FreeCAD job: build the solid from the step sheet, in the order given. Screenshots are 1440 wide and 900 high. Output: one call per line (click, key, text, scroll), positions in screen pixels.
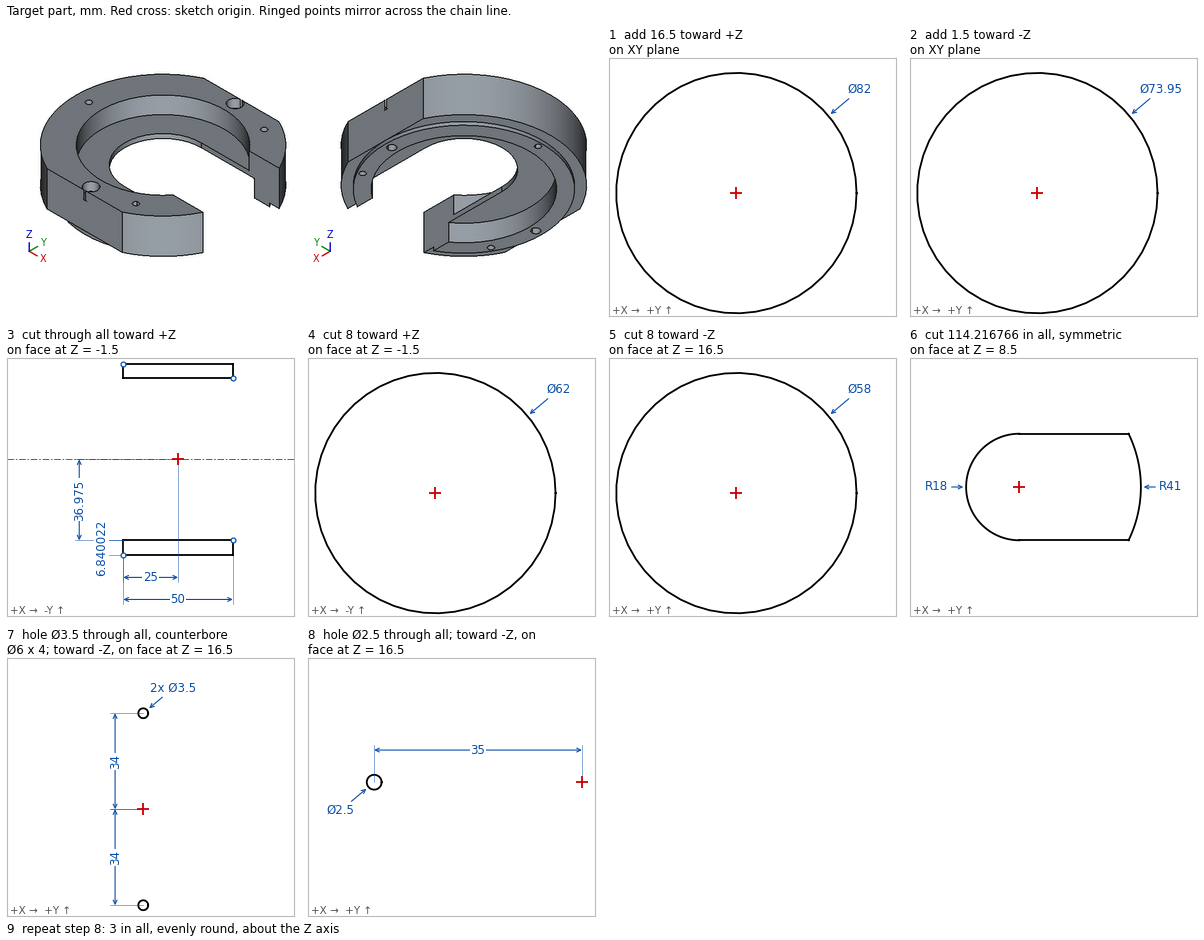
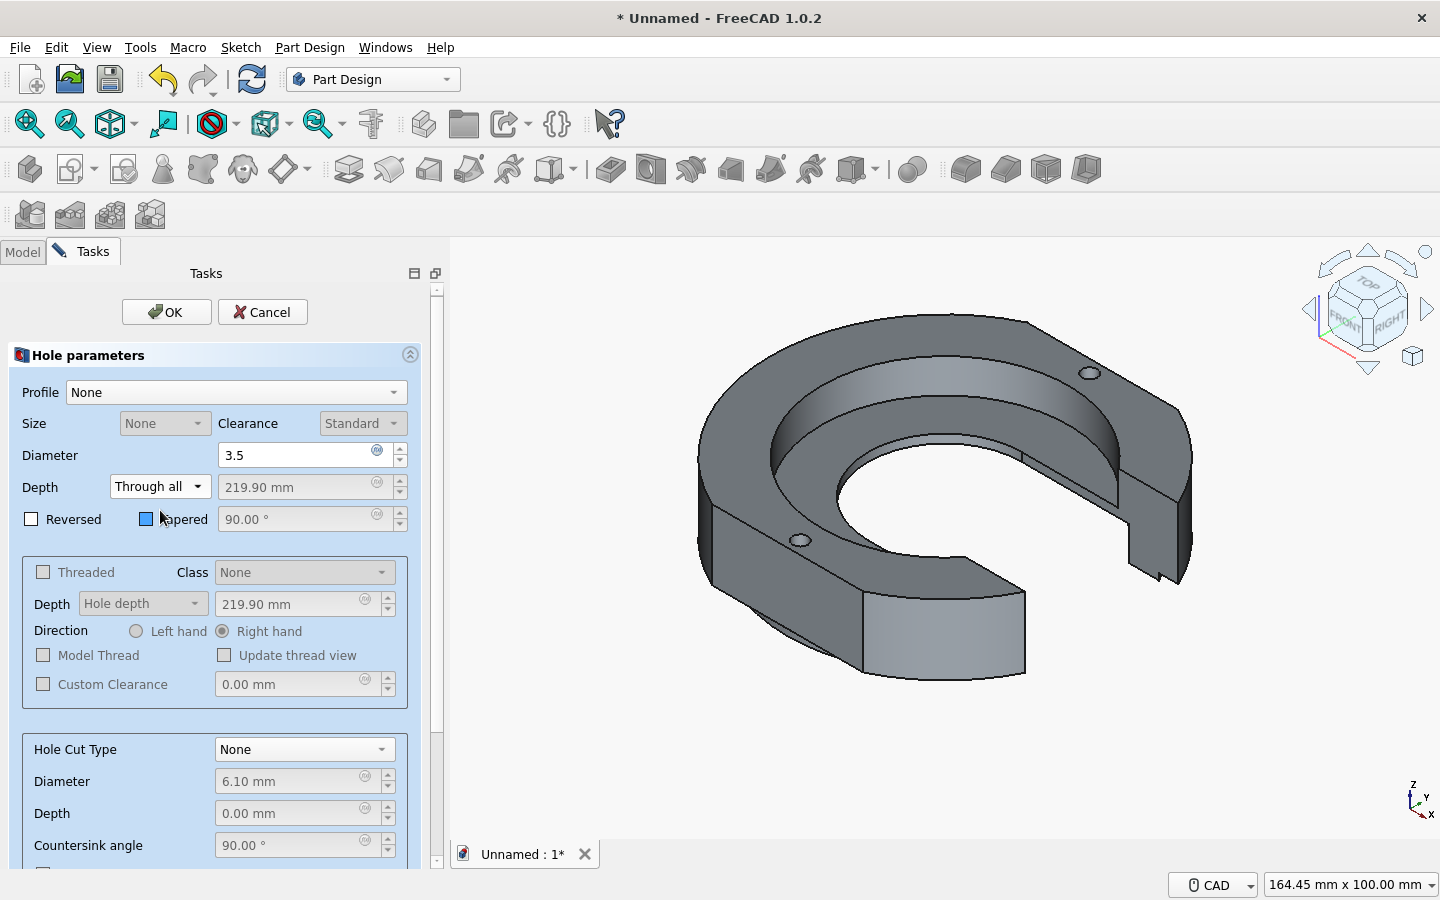
click(306, 750)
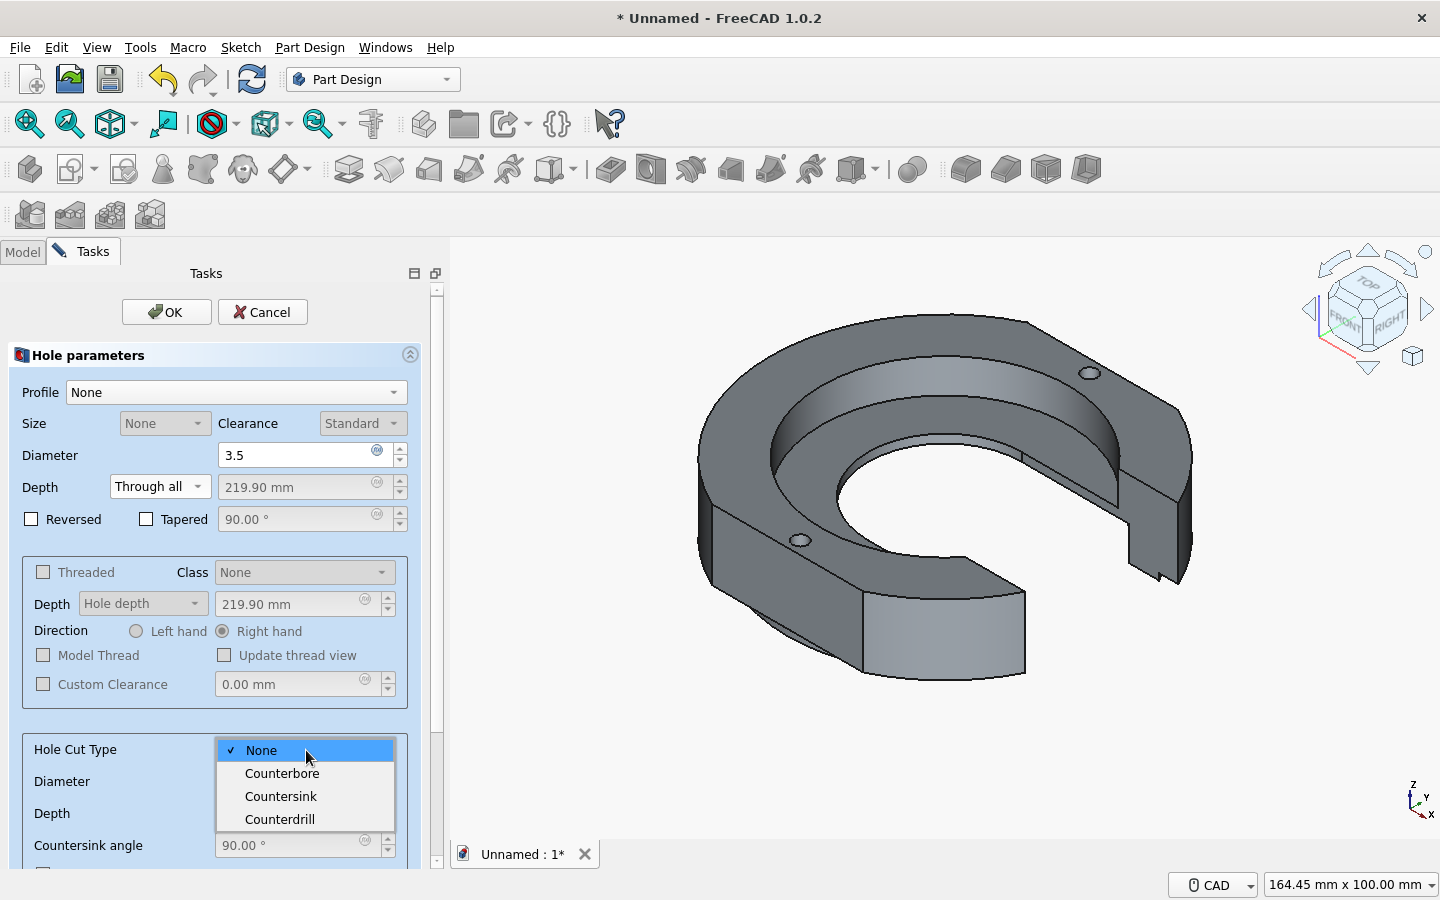
click(304, 774)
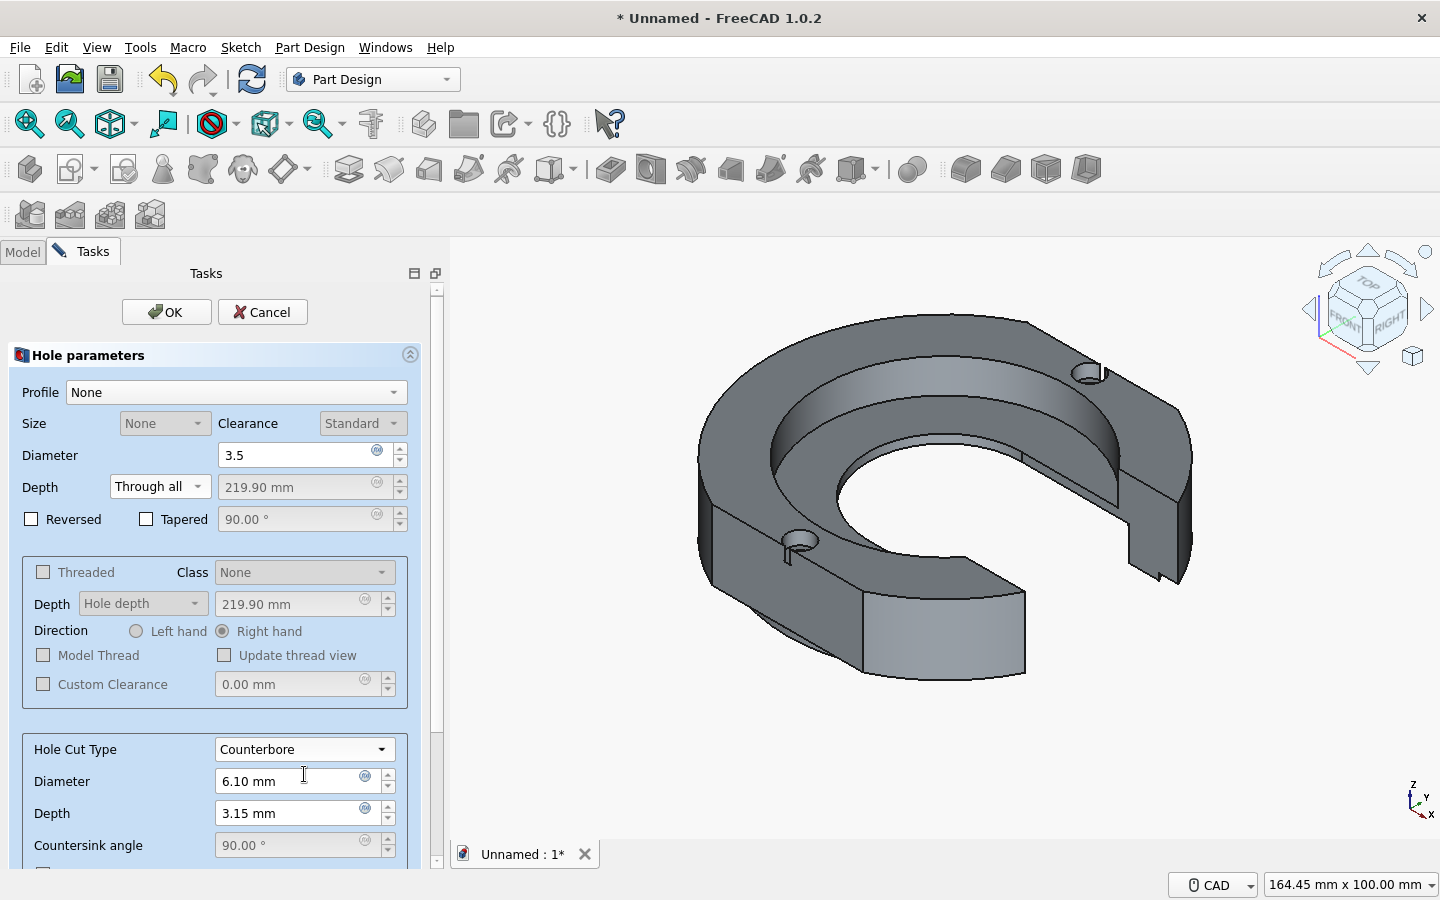
triple_click(298, 781)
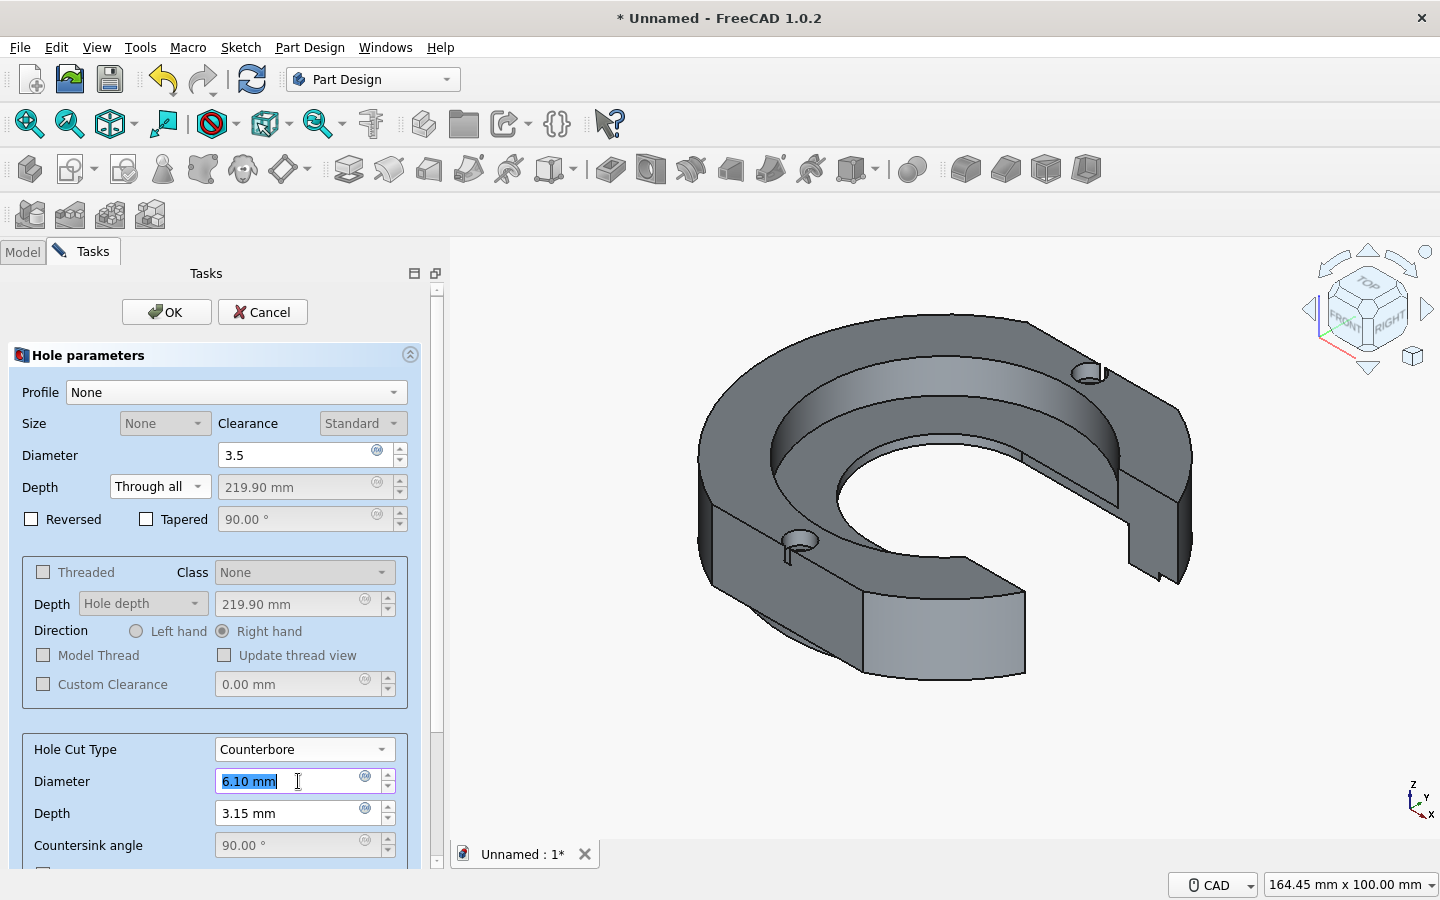
text(6)
key(Tab)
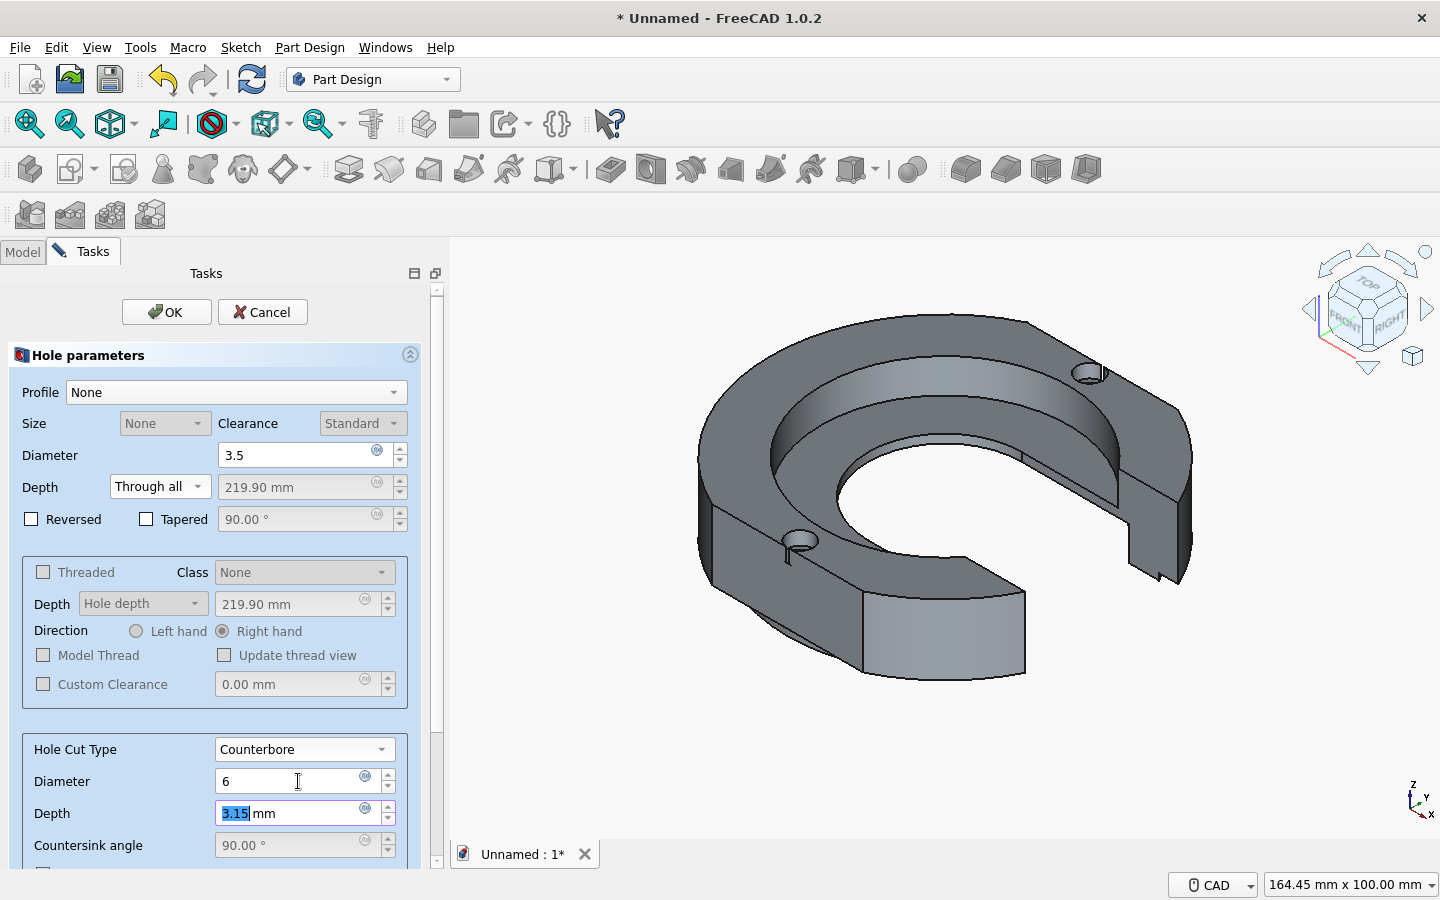
text(4)
key(Tab)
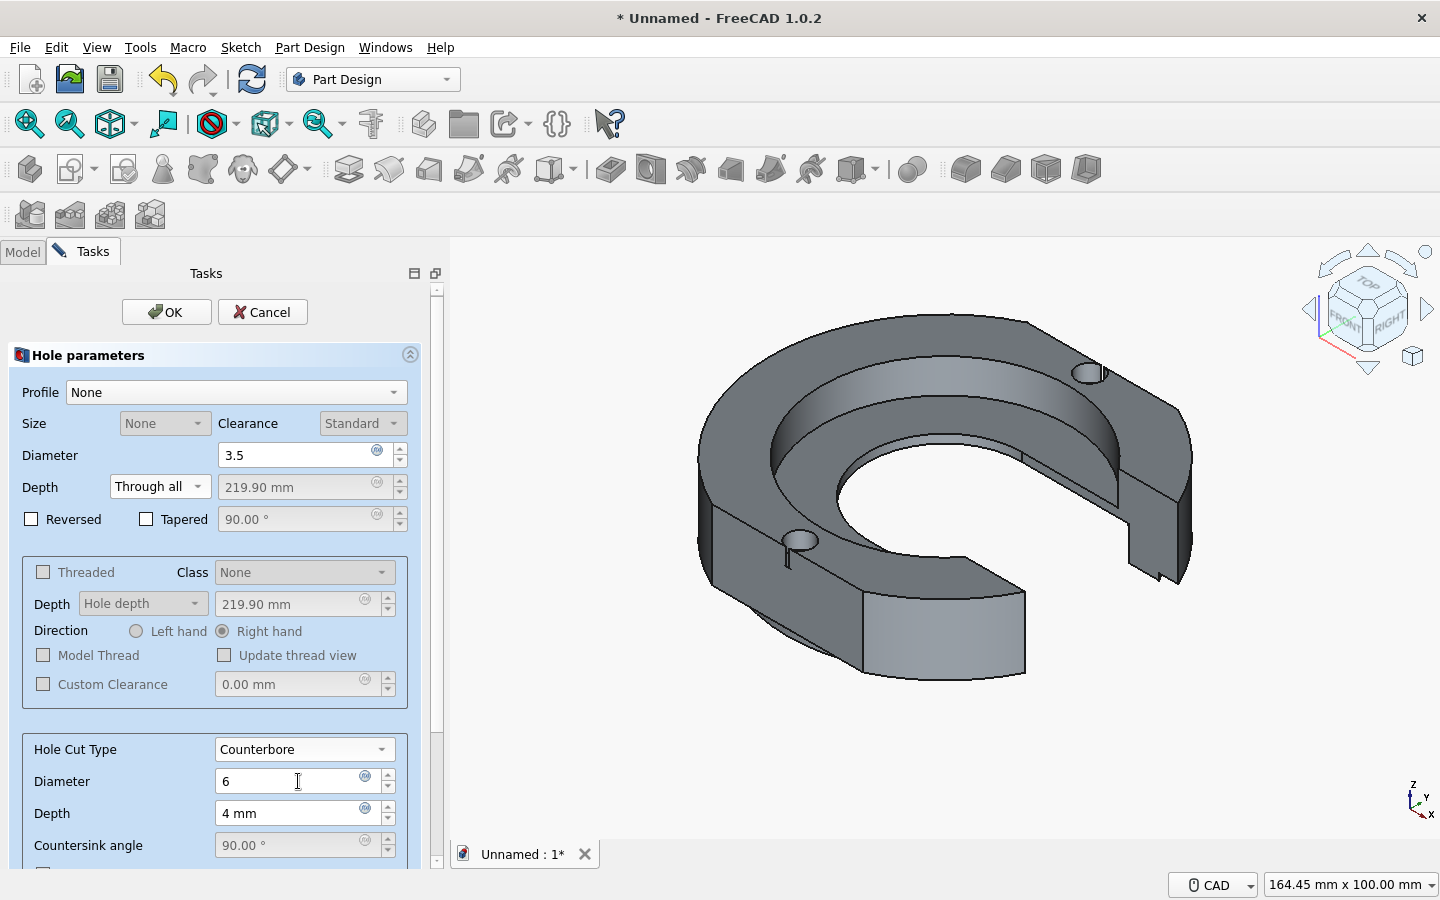
click(167, 312)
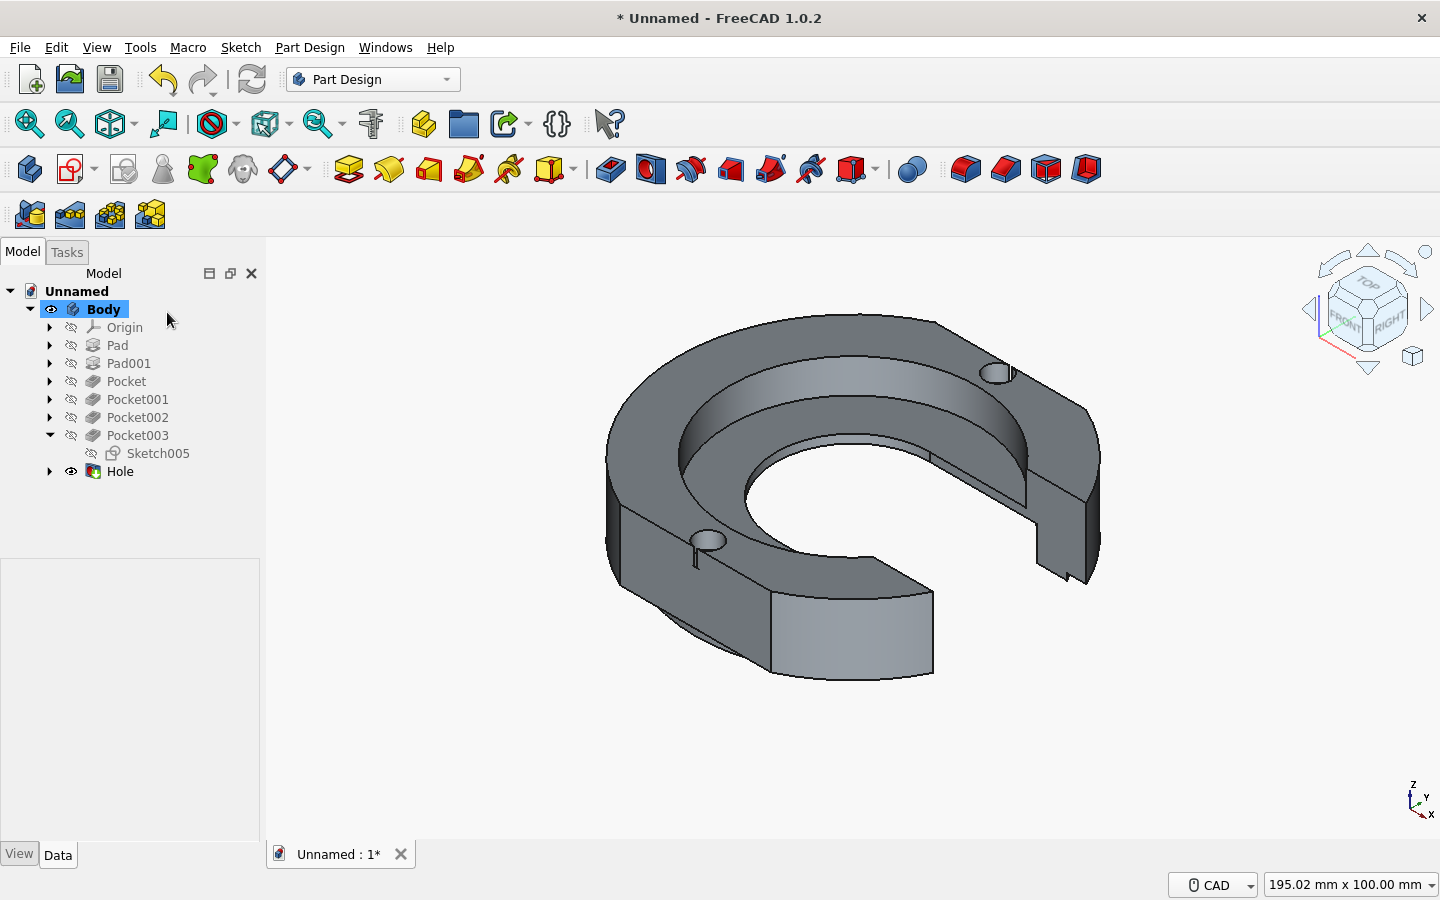
click(702, 369)